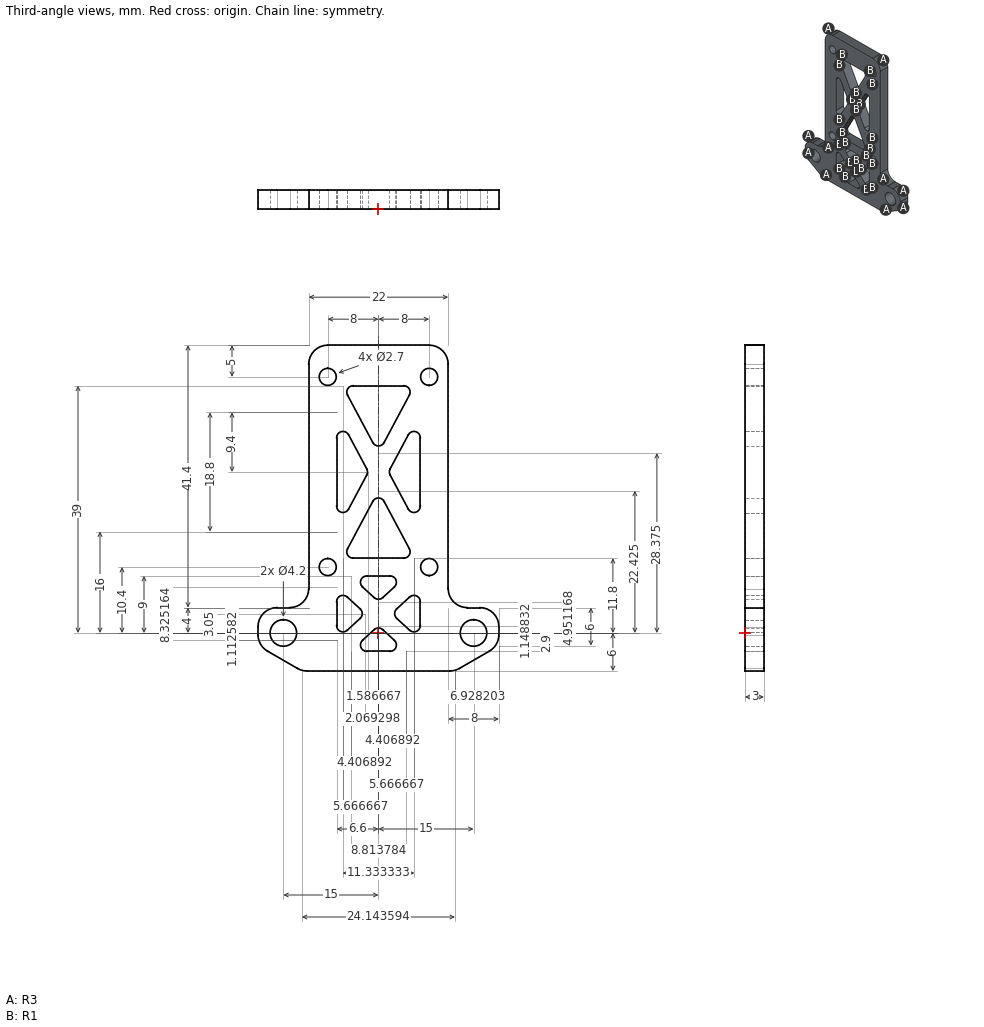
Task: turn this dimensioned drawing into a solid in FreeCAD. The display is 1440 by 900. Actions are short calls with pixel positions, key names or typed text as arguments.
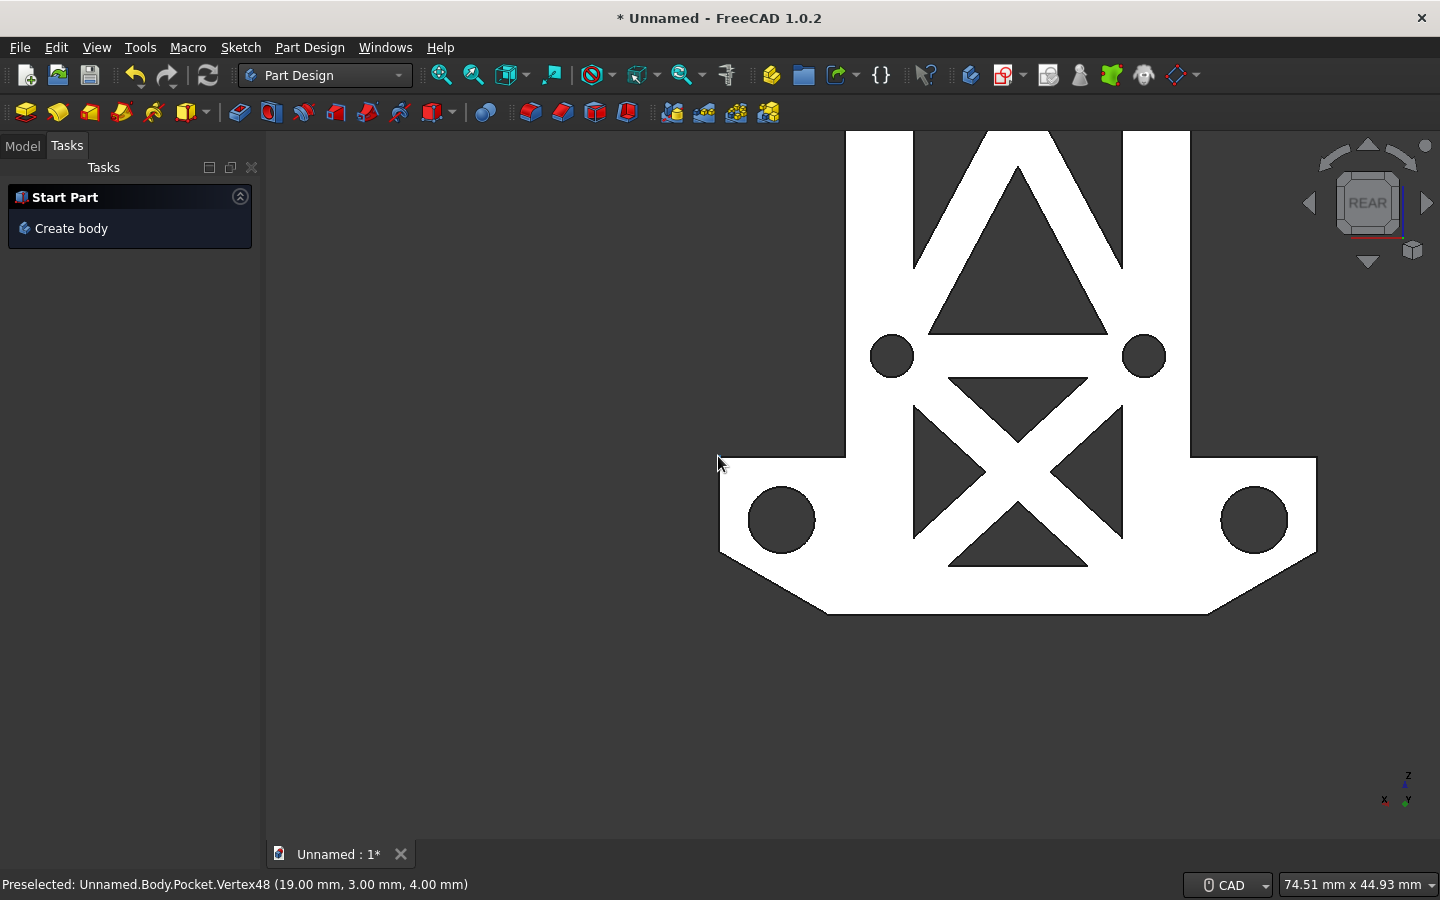
click(442, 76)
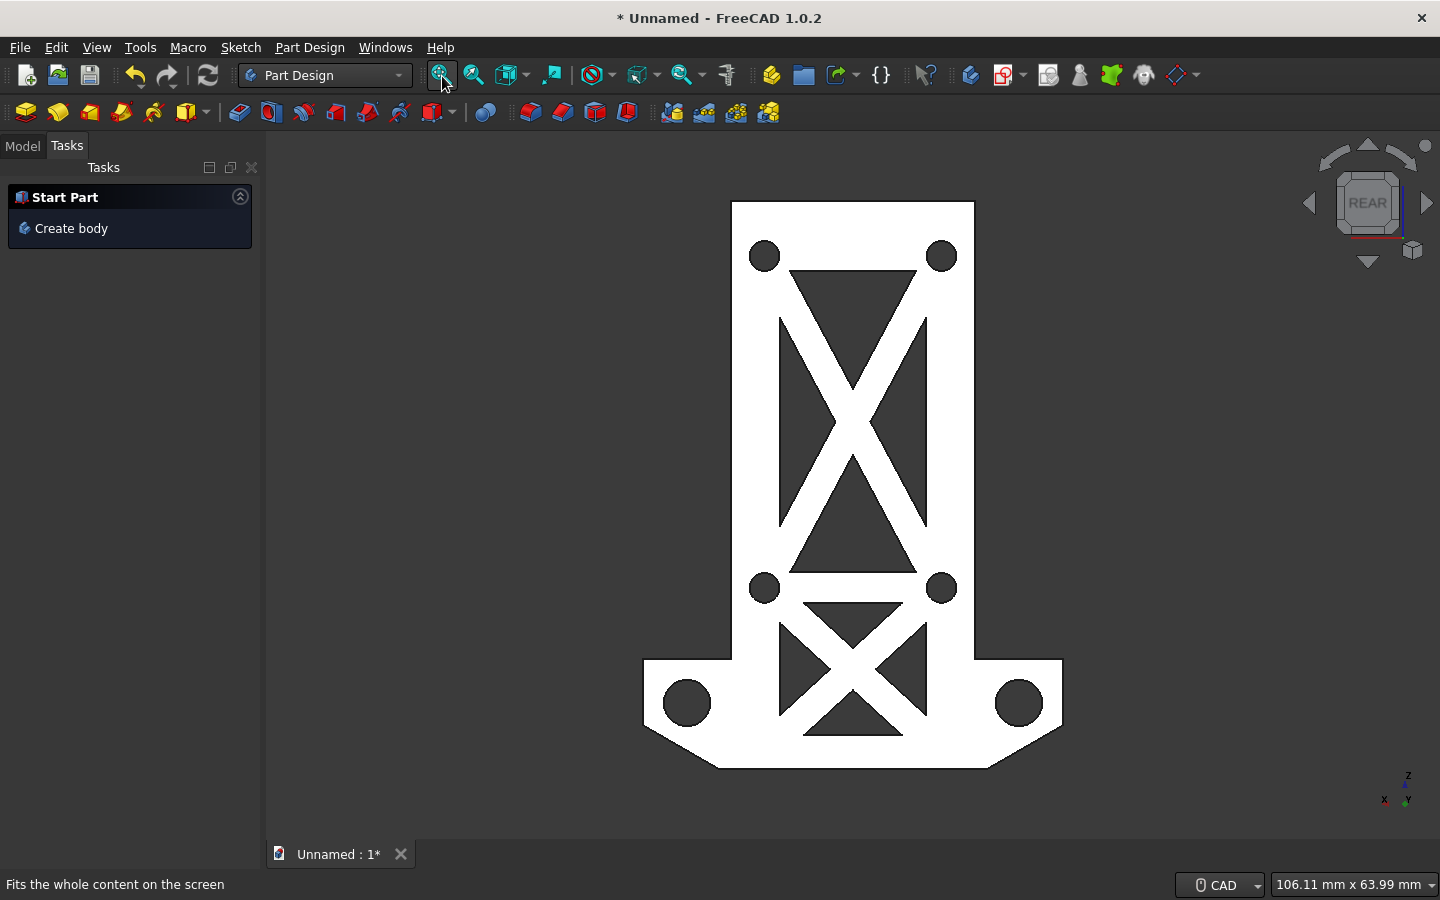
key(0)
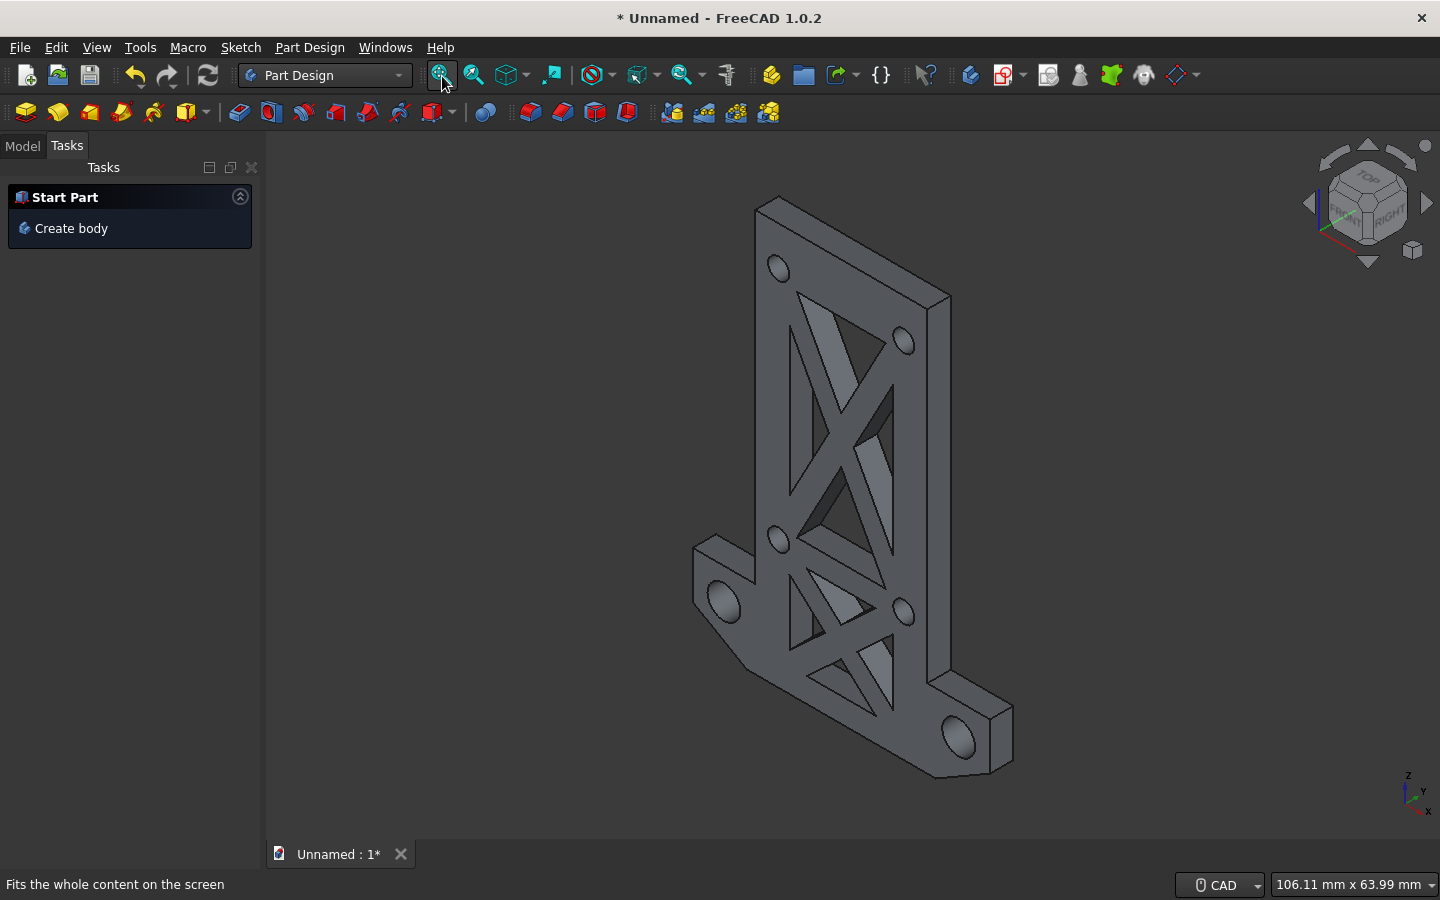
click(1002, 712)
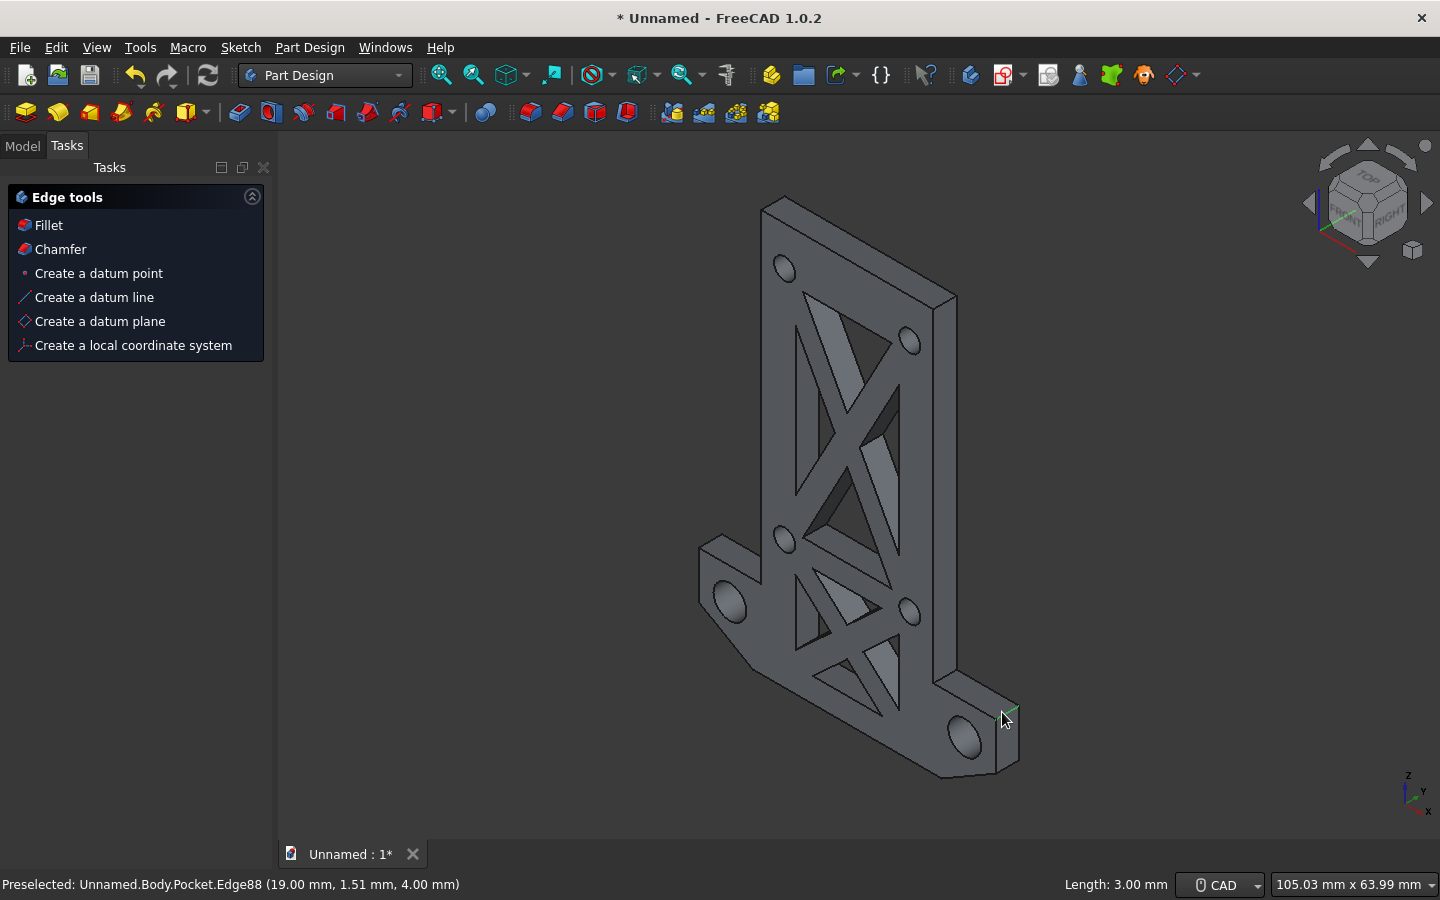
click(945, 302, ctrl)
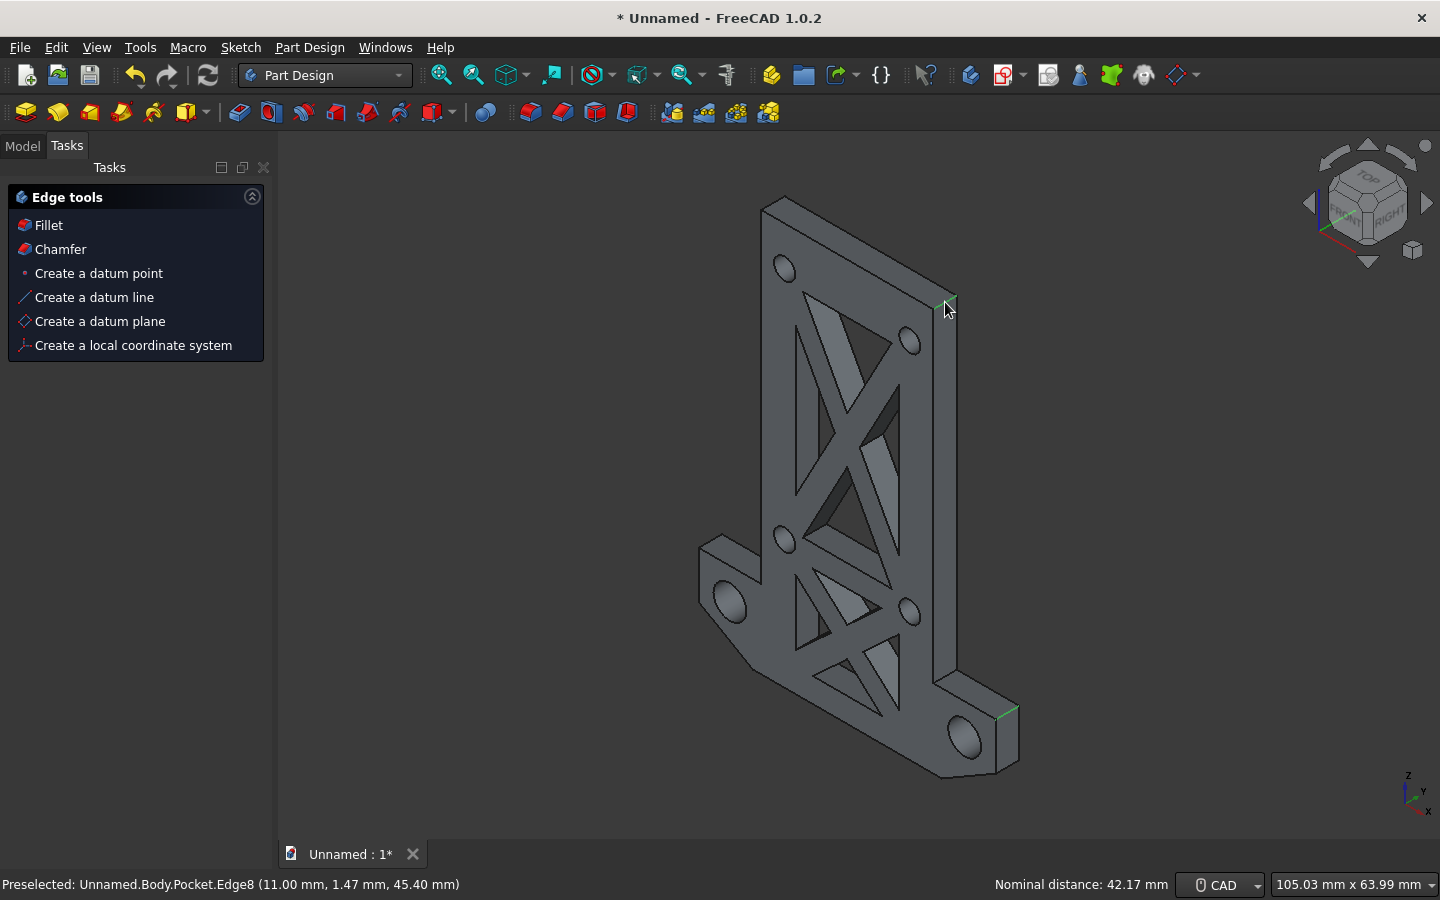
key(2)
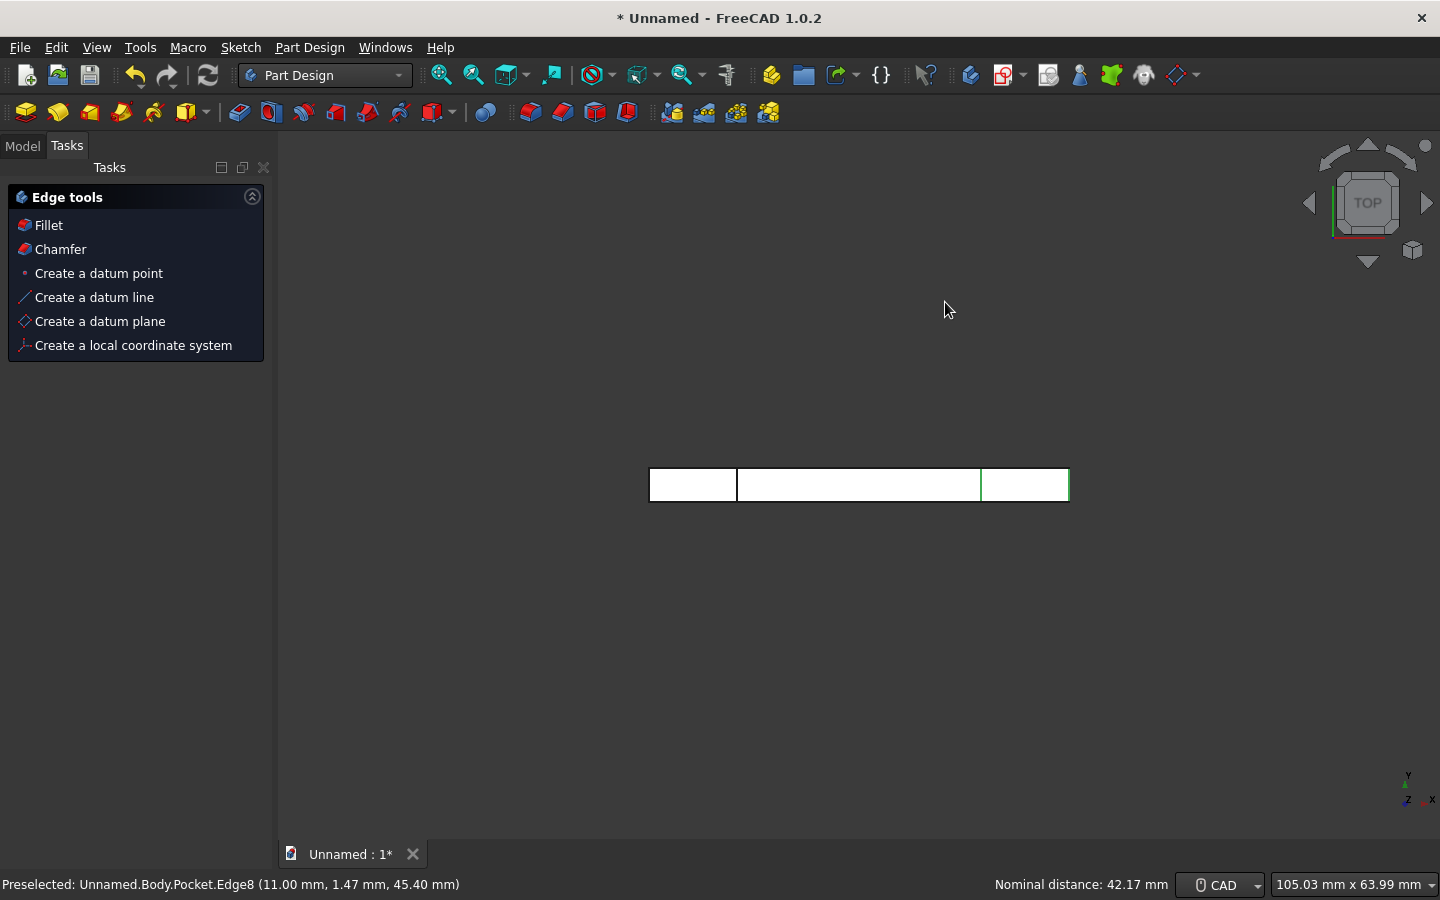
click(442, 76)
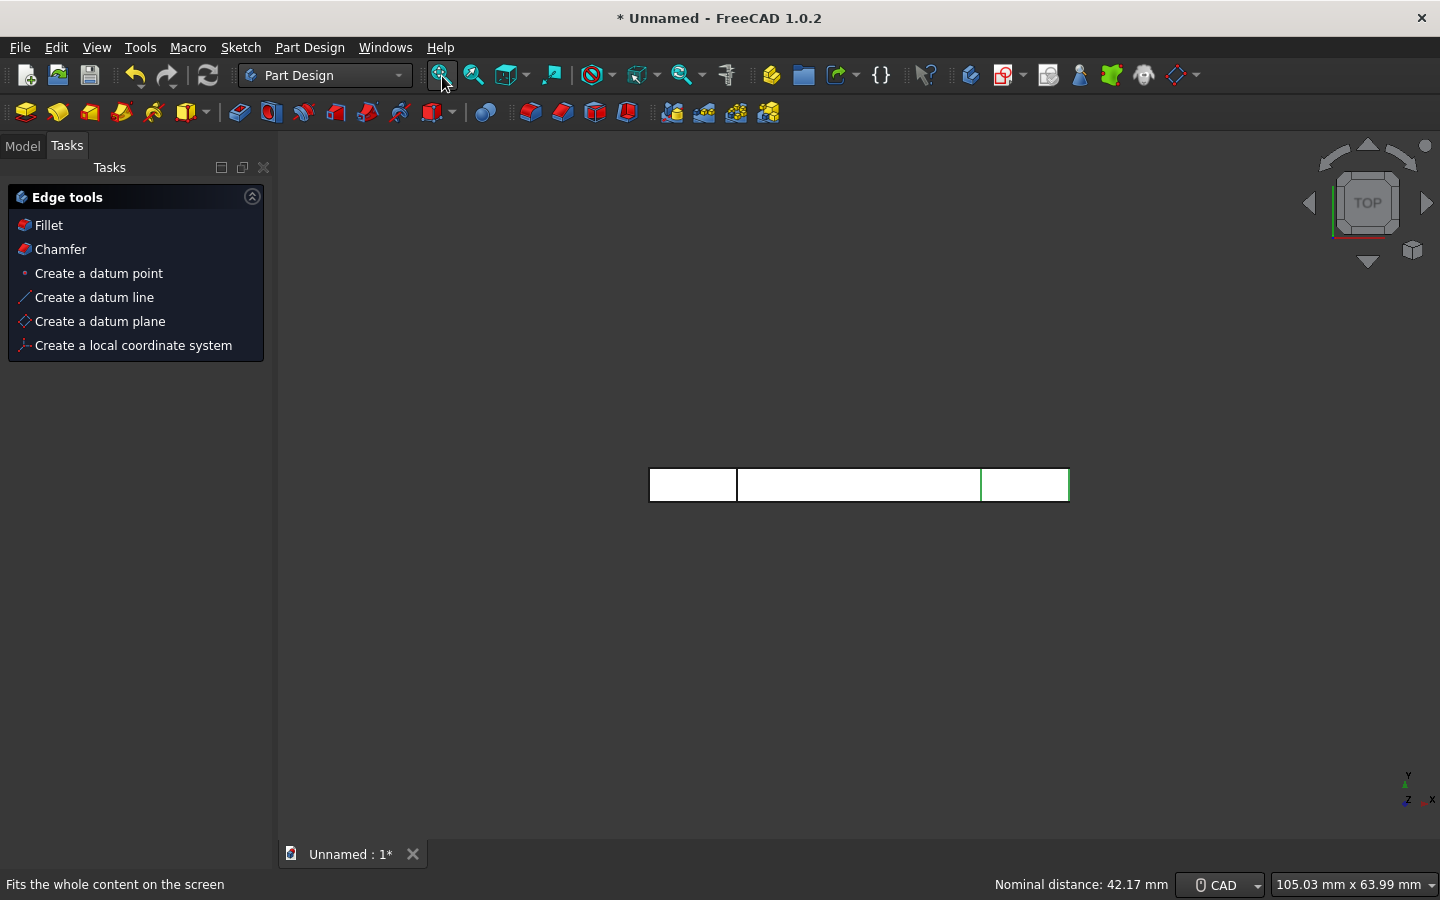
click(737, 484, ctrl)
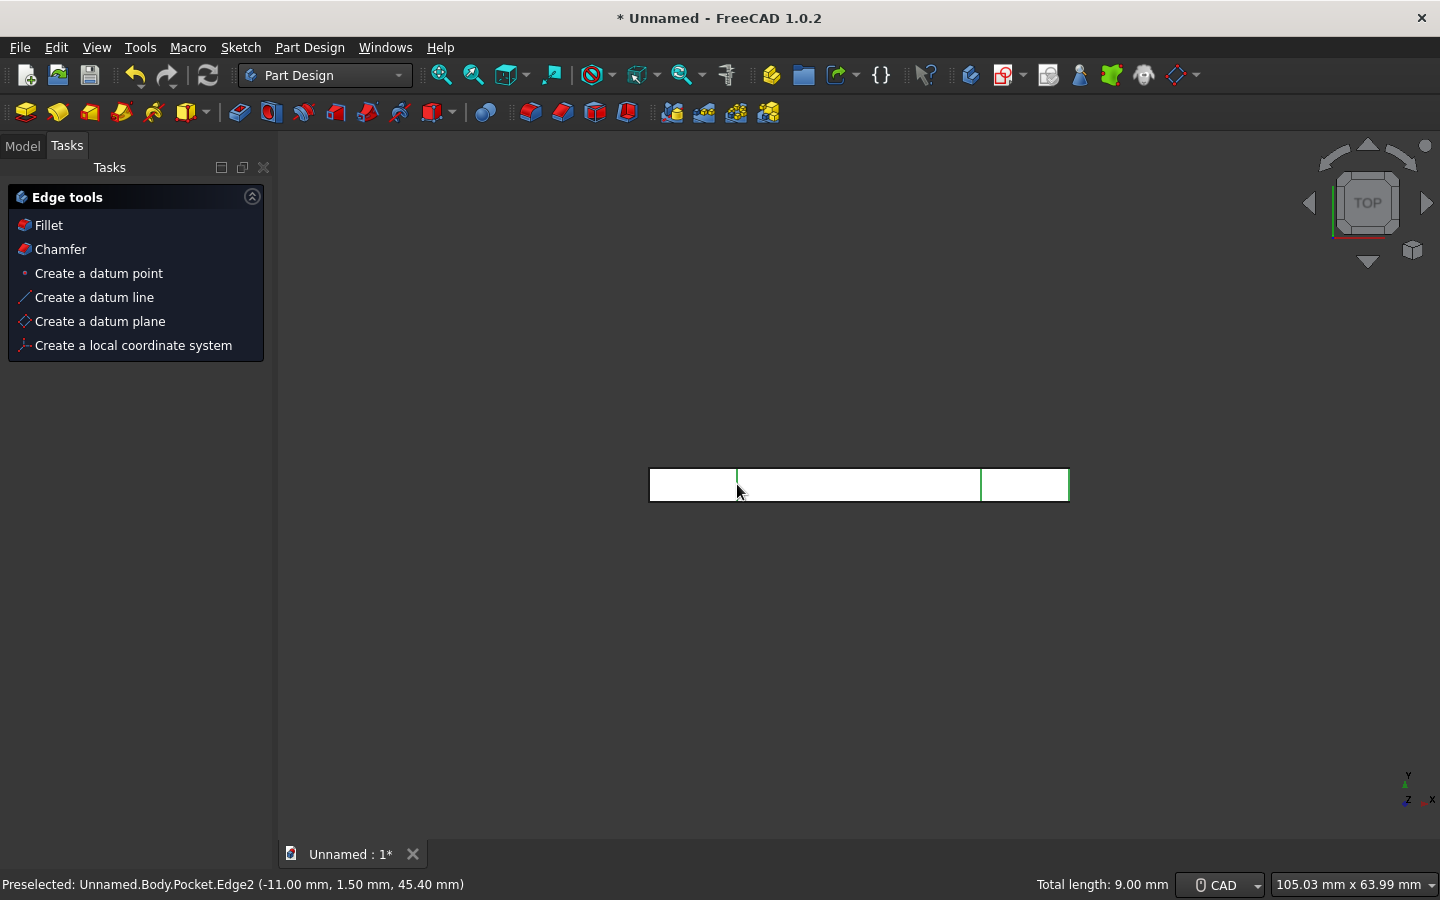
click(649, 484, ctrl)